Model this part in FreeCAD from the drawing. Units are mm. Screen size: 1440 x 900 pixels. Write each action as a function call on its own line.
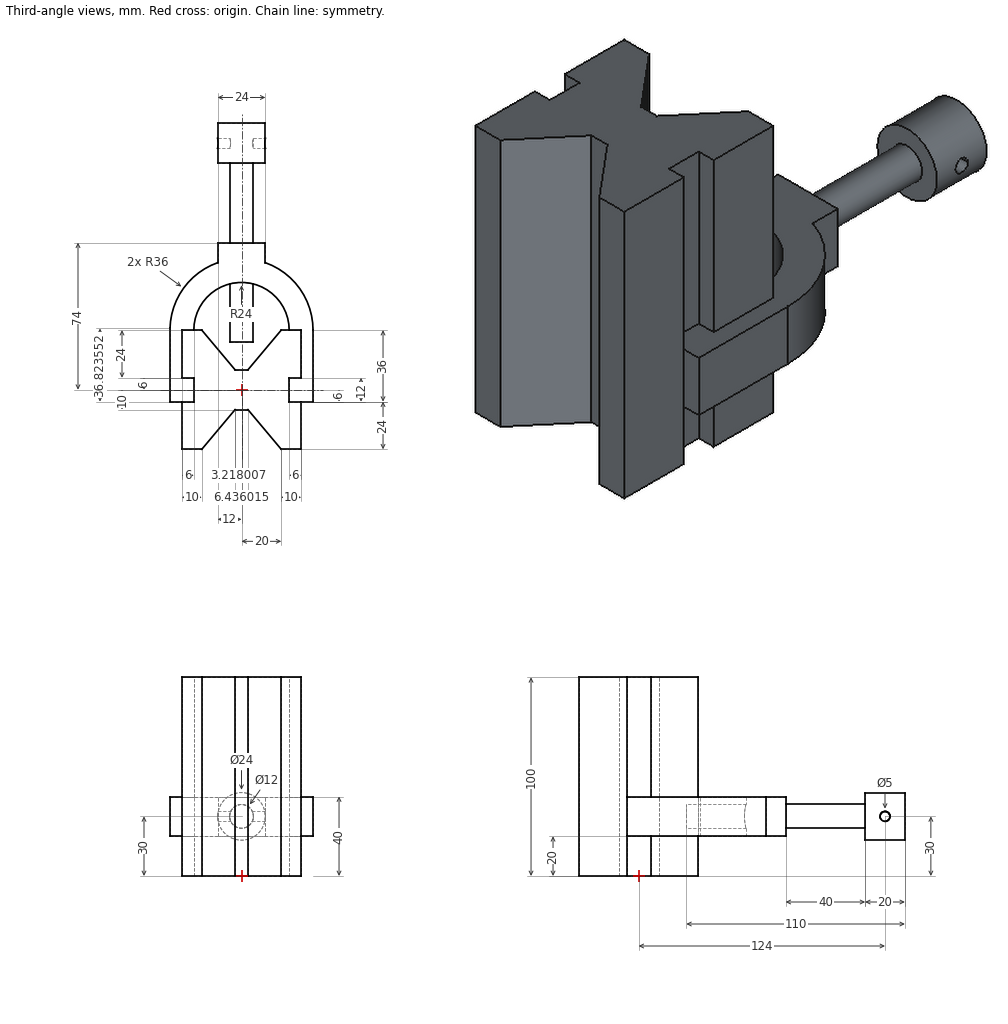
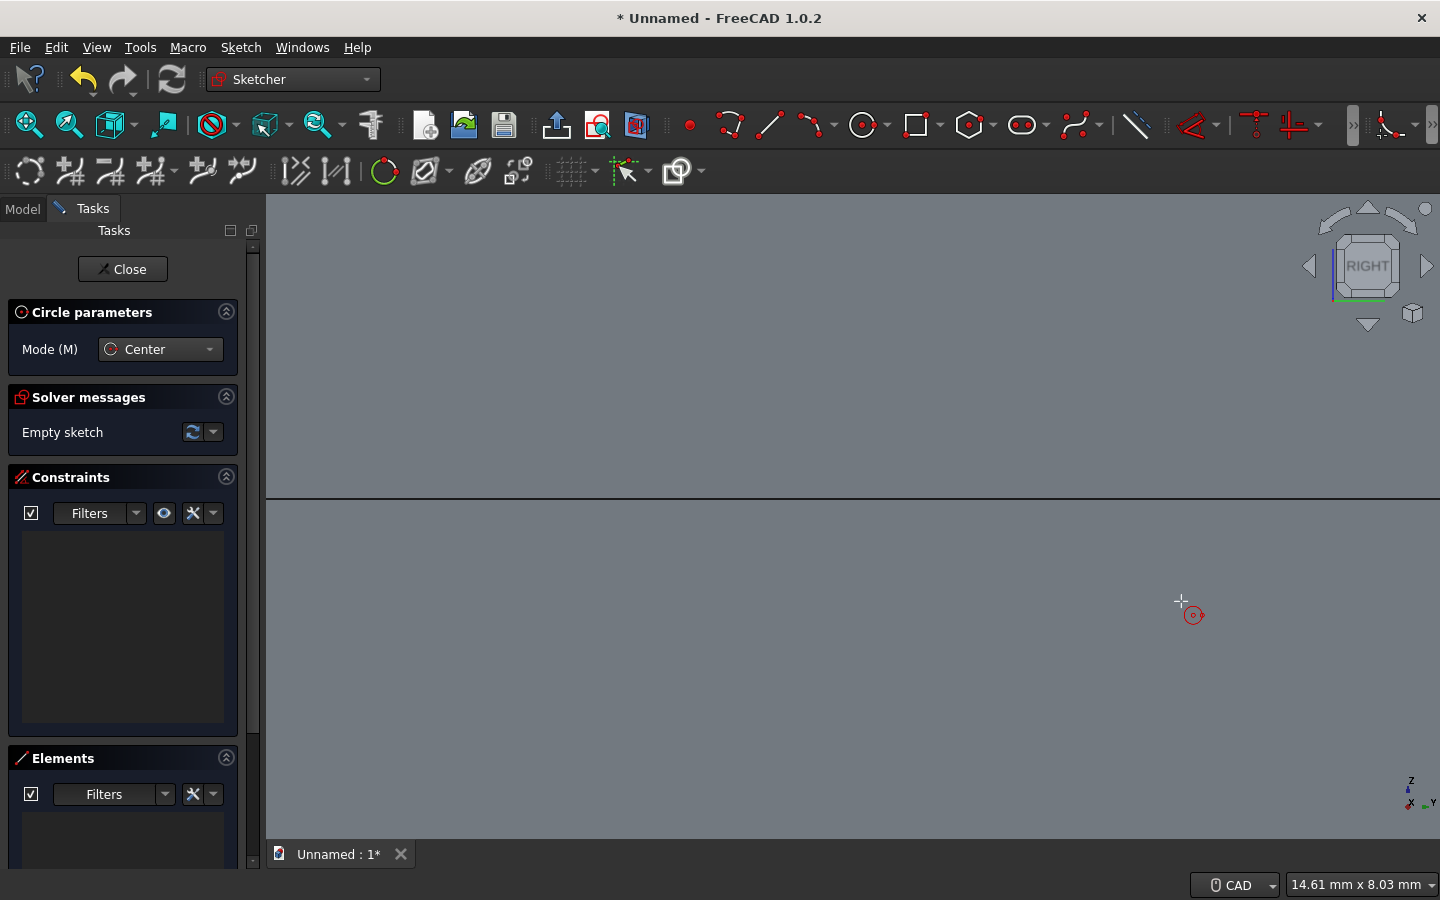
click(765, 499)
move(907, 357)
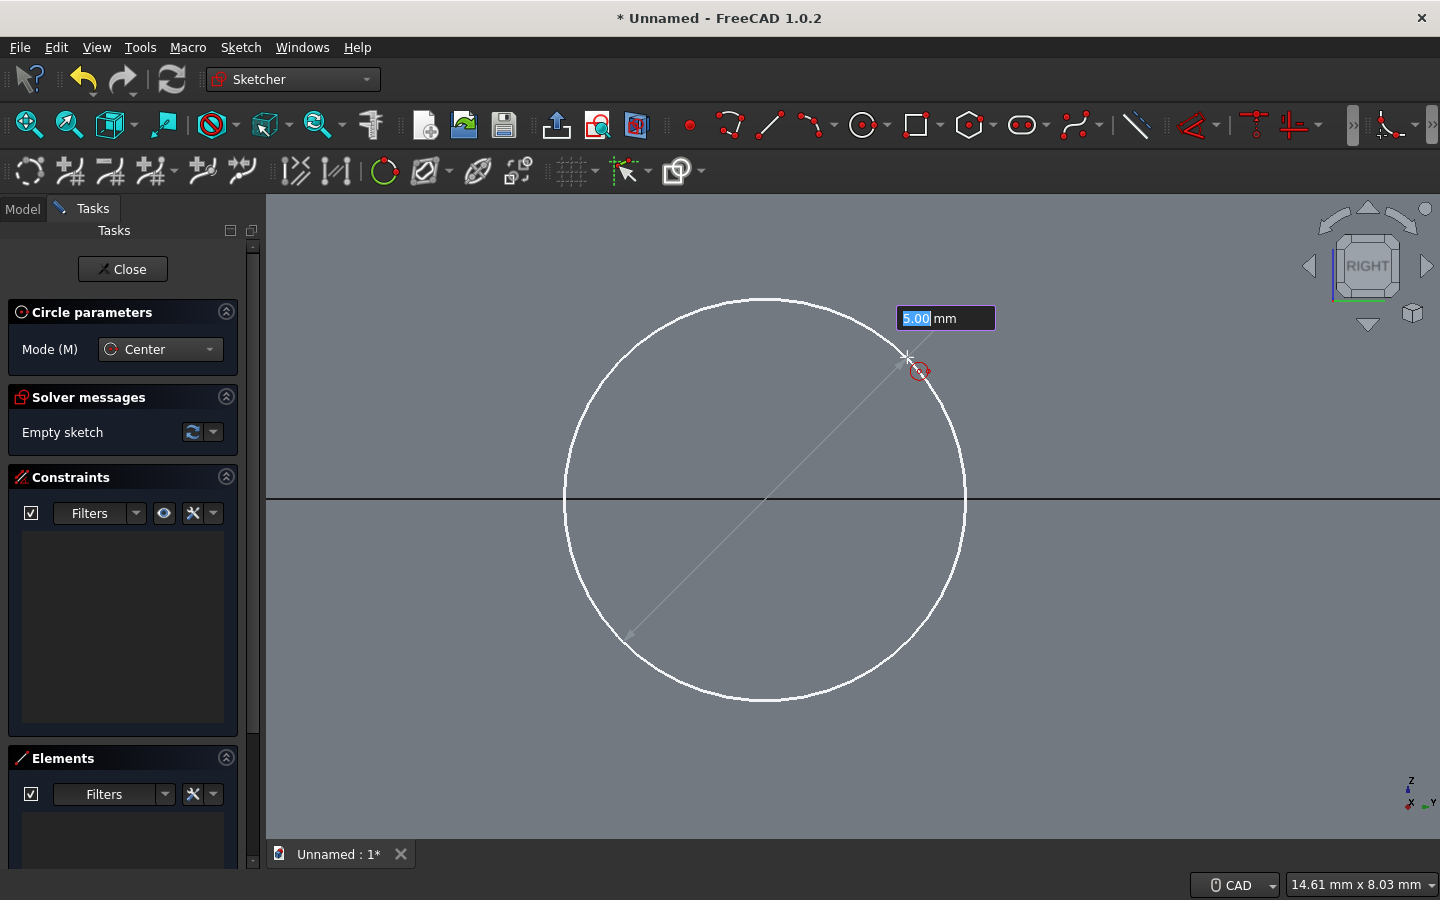
text(5)
key(Return)
key(Escape)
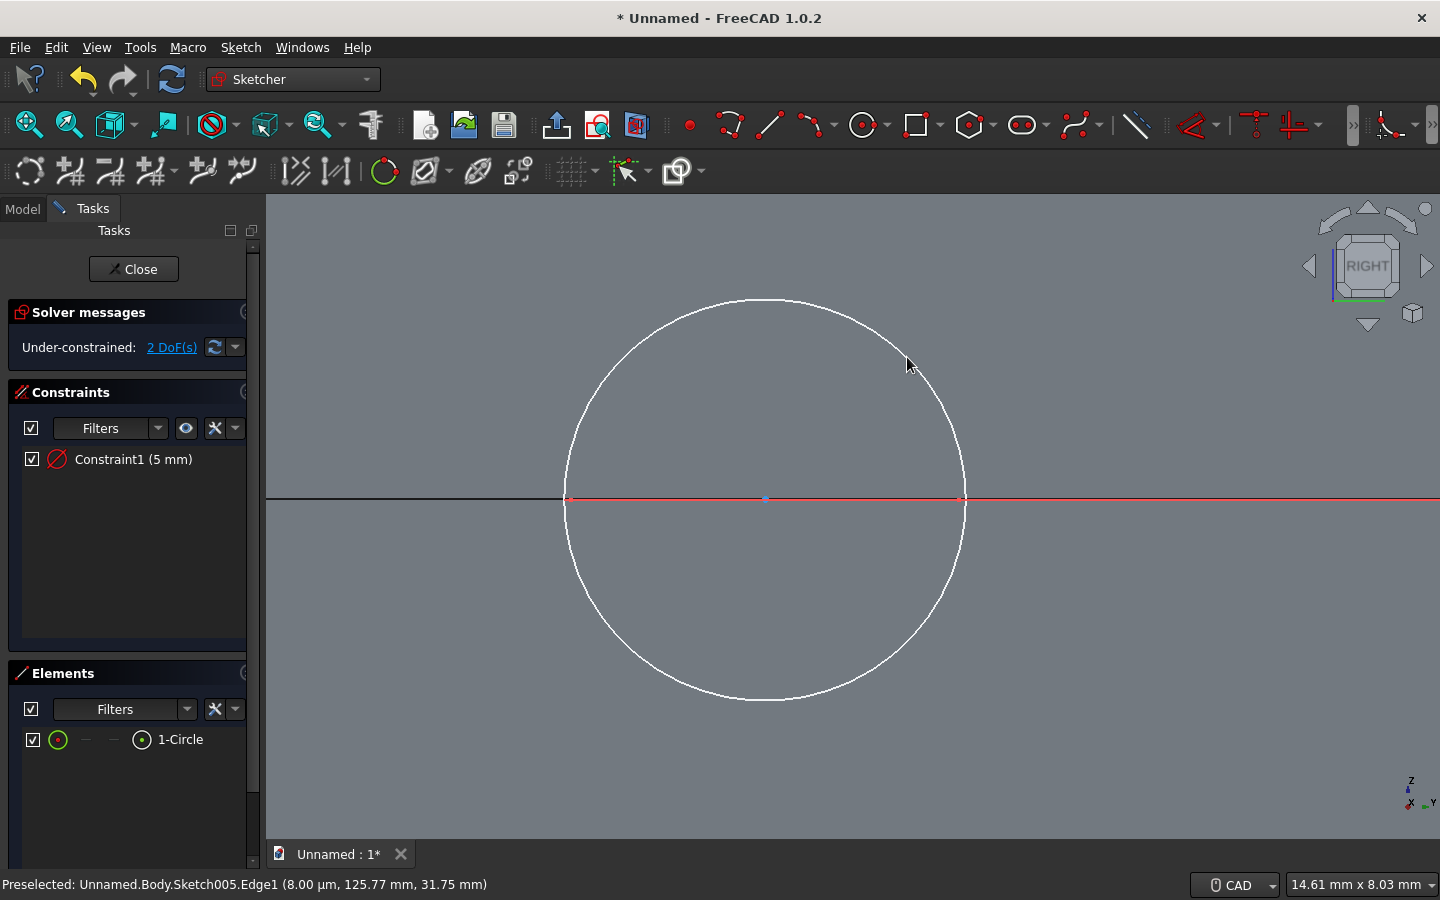
click(1192, 126)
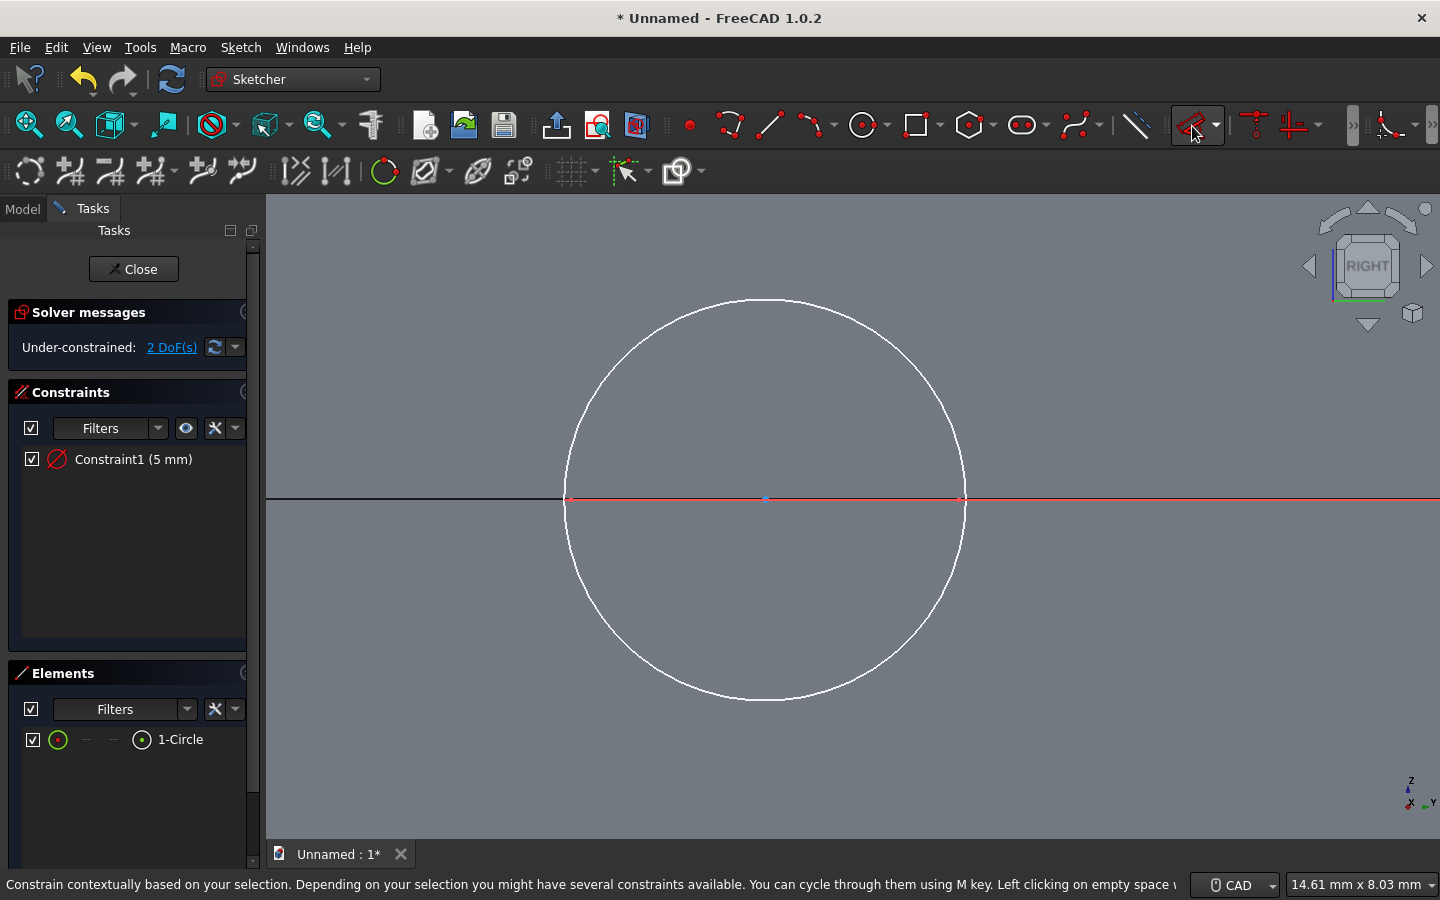
click(765, 500)
click(799, 655)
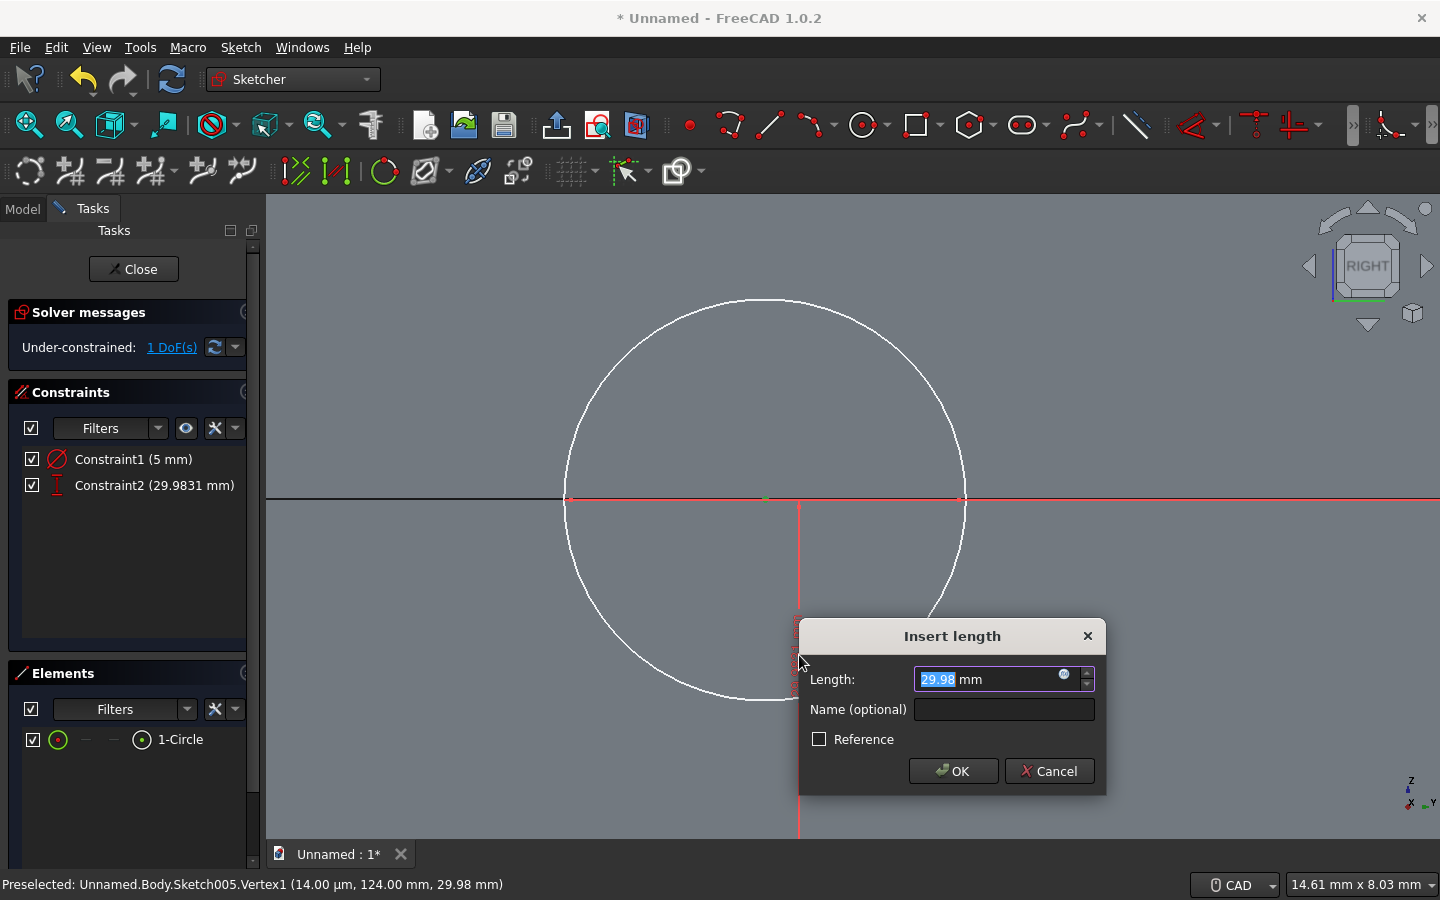
text(30)
key(Return)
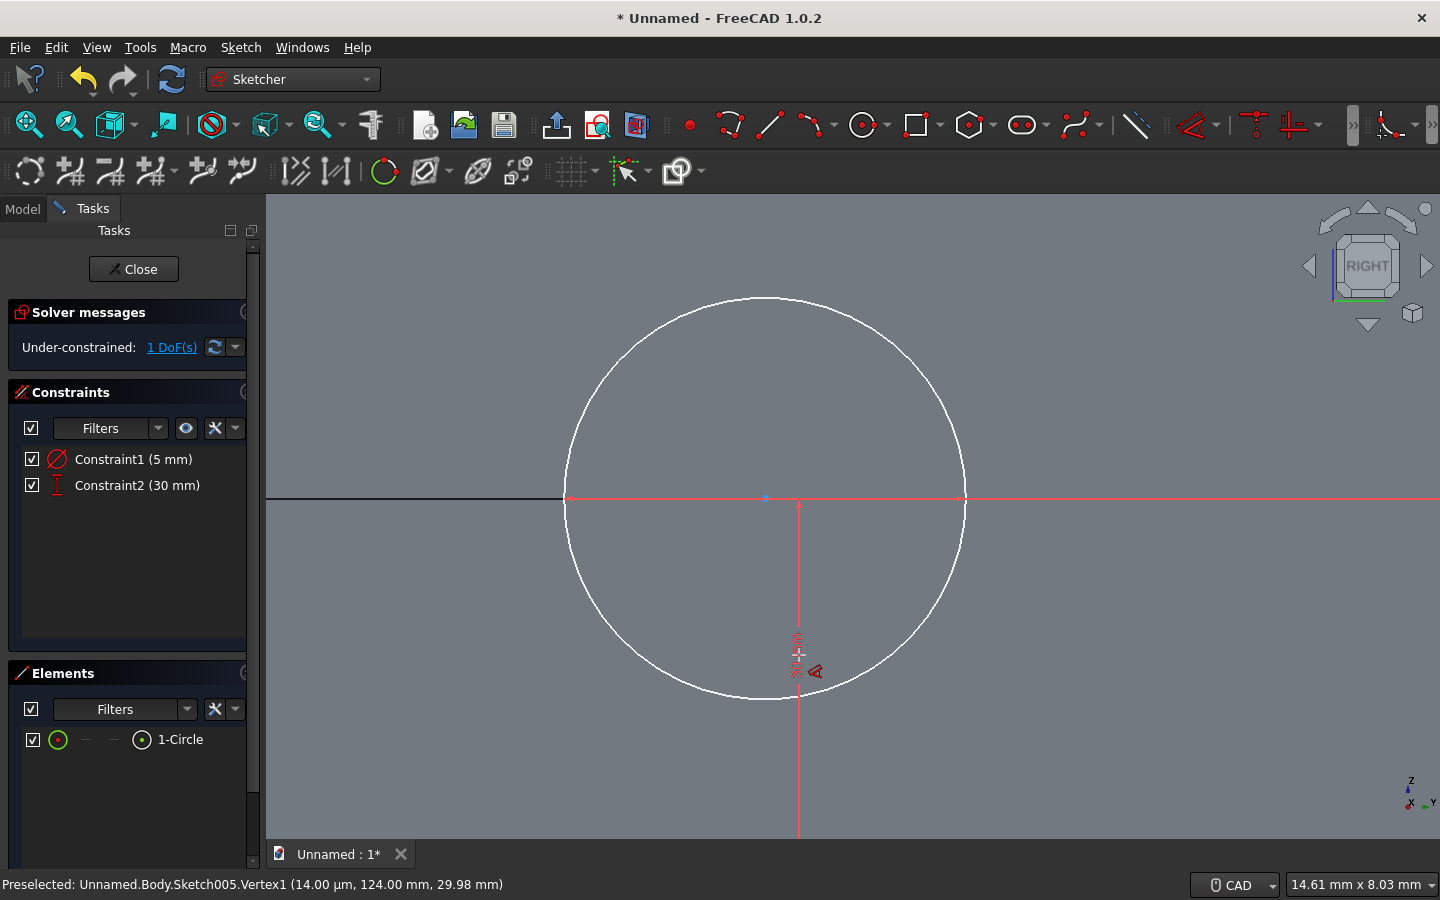
click(765, 499)
click(530, 465)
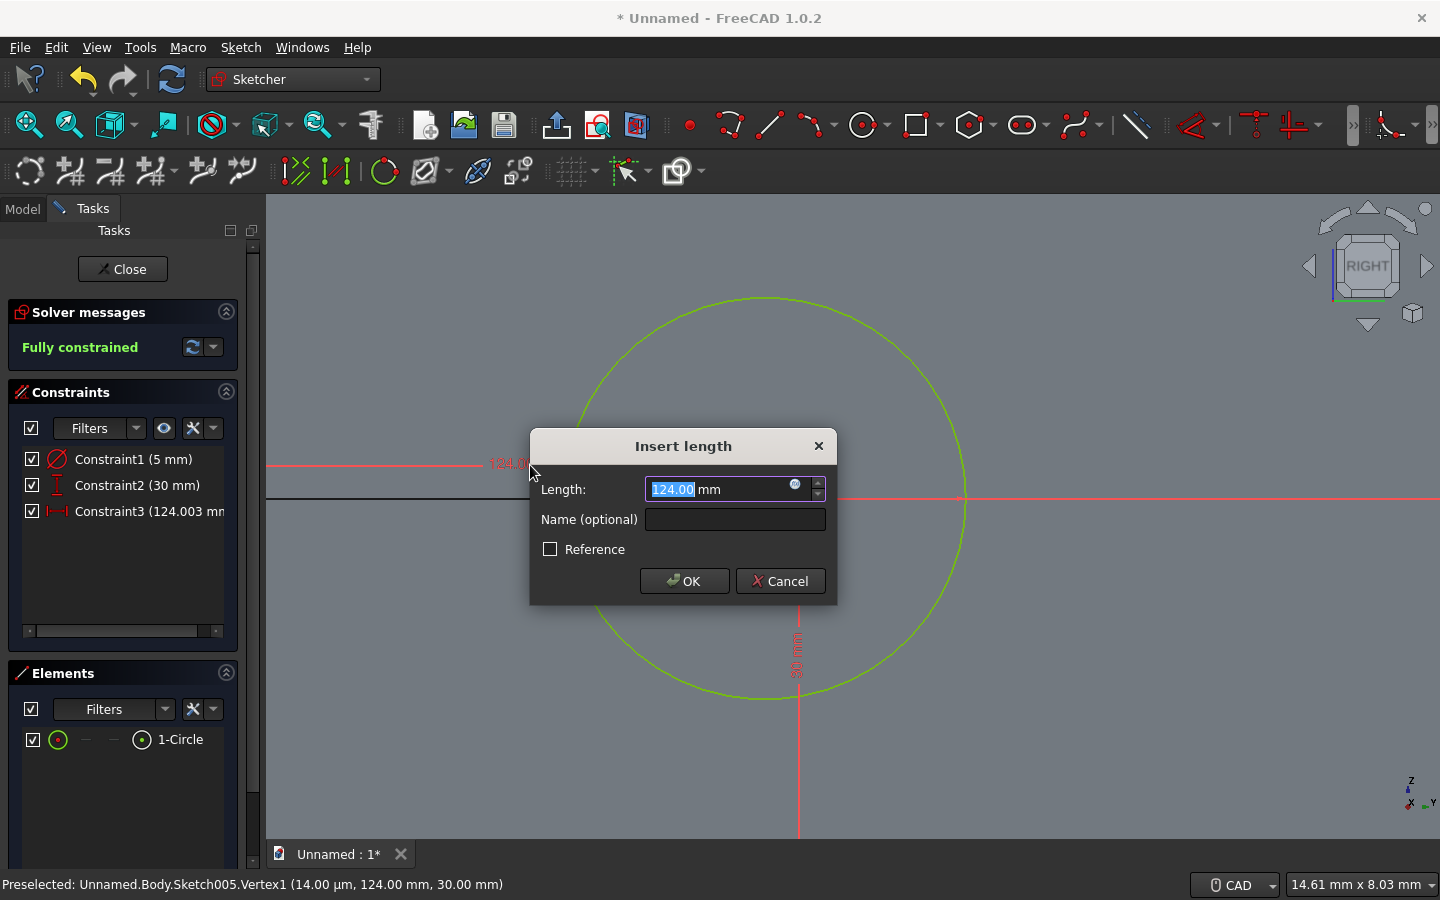
text(124)
key(Return)
key(Escape)